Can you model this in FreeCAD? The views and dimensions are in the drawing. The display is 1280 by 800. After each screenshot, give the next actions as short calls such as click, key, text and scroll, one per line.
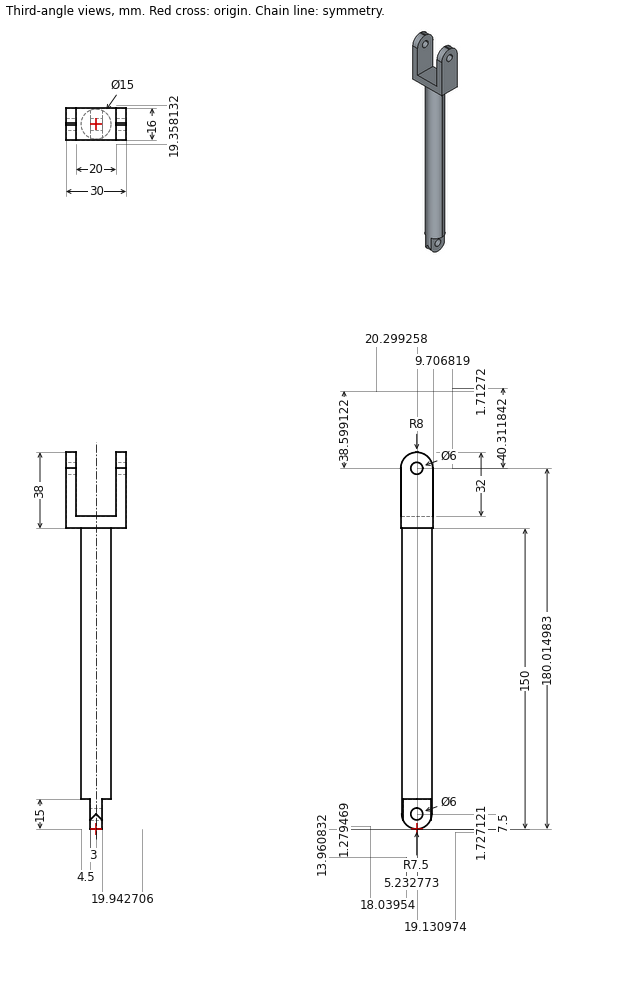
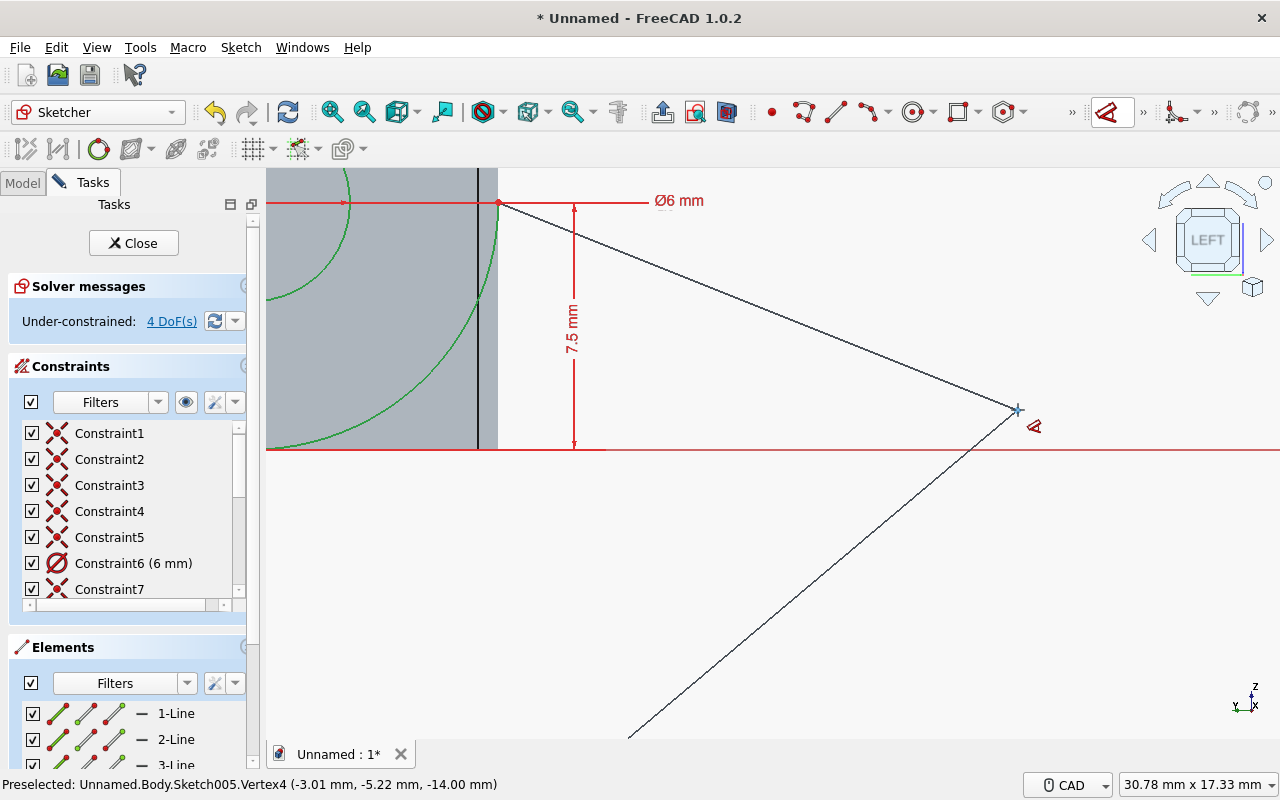
click(1017, 410)
click(1051, 430)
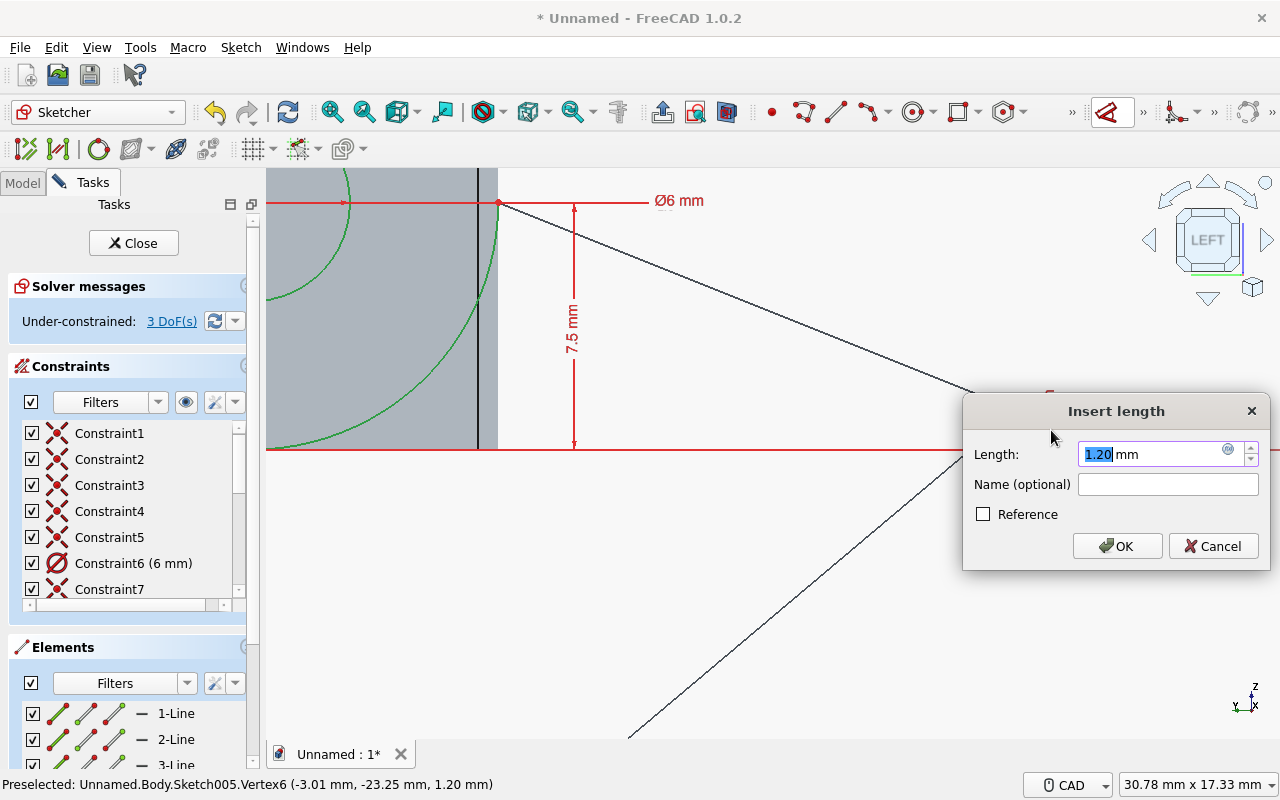
text(1.279469)
key(Return)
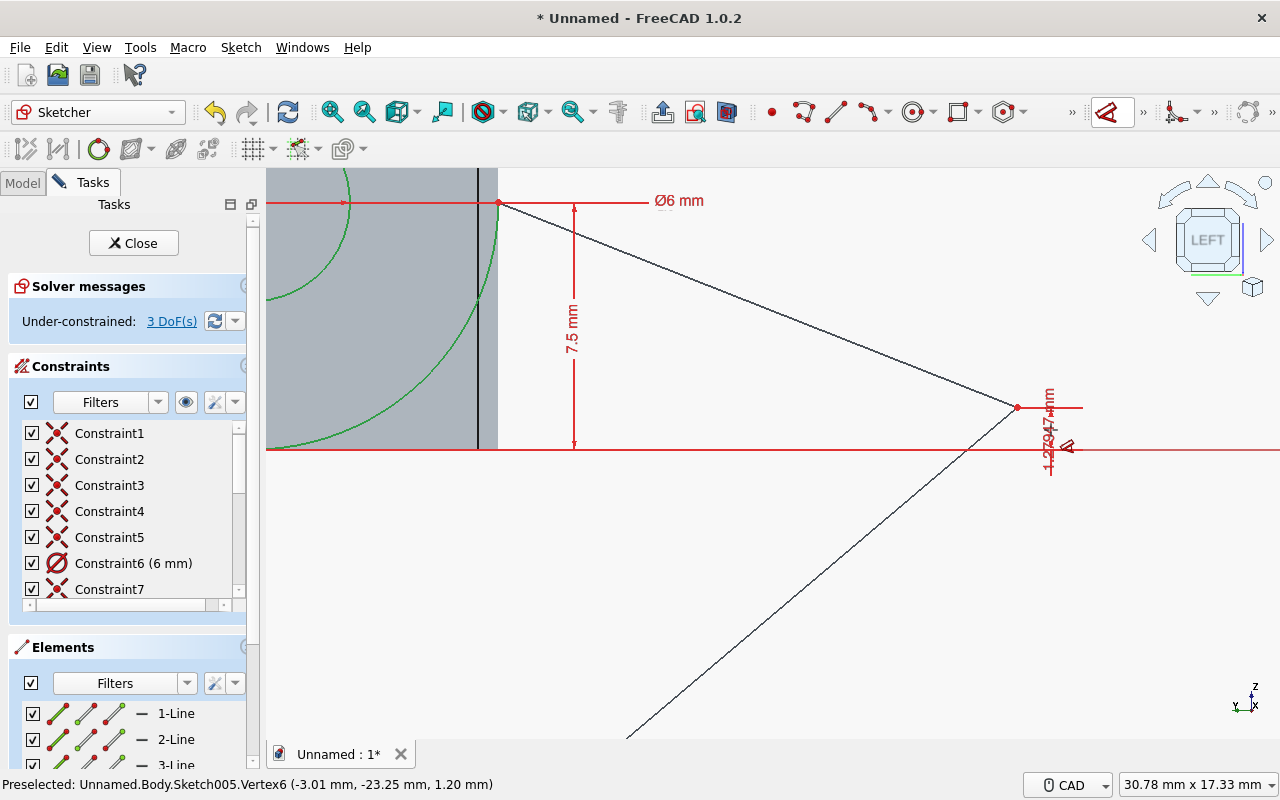
click(839, 559)
click(720, 374)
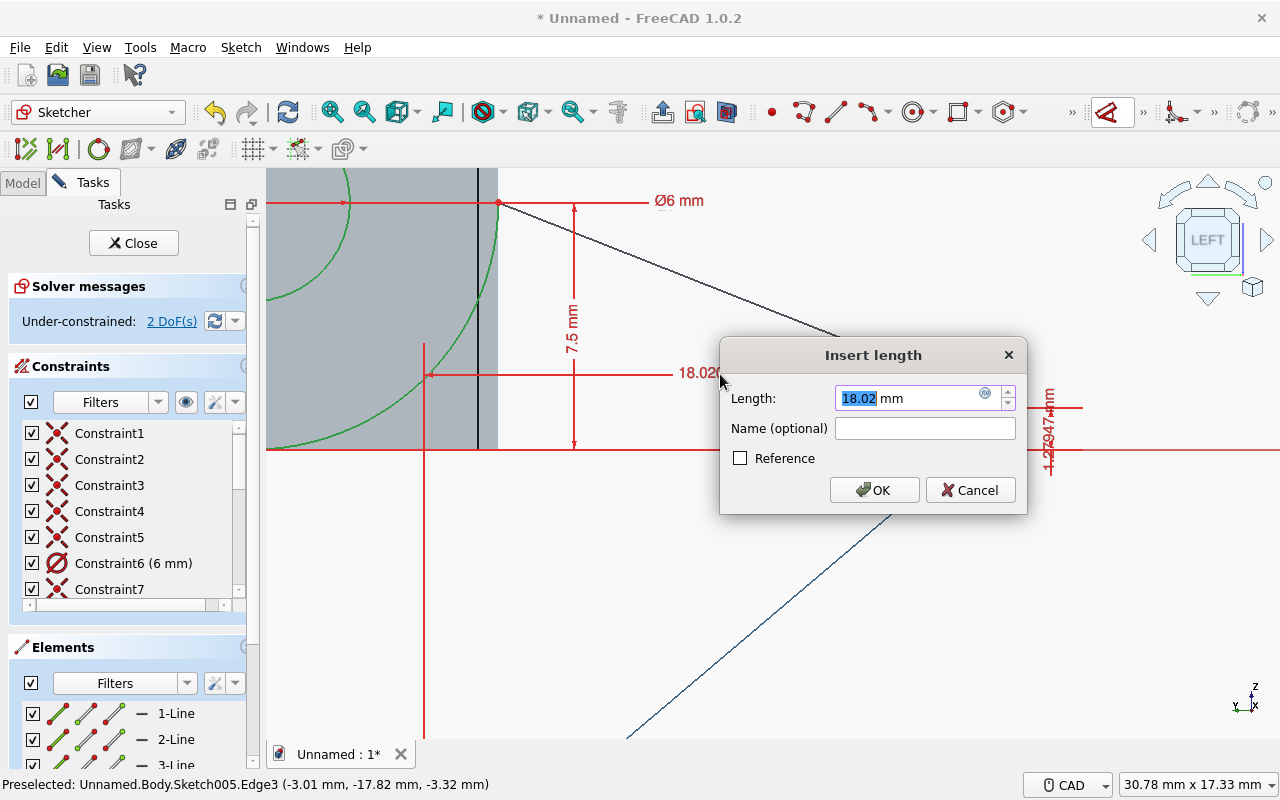
text(18.03954)
key(Return)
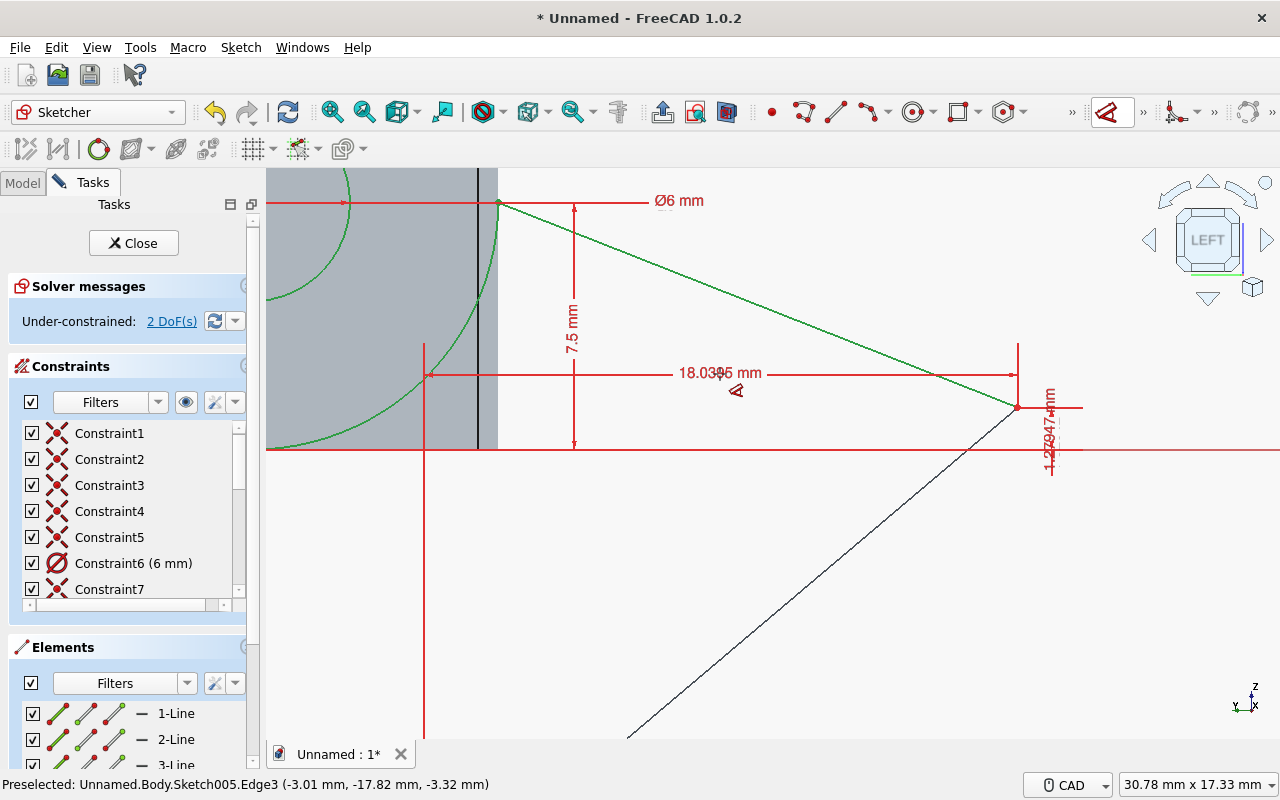
scroll(1019, 410, down, 4)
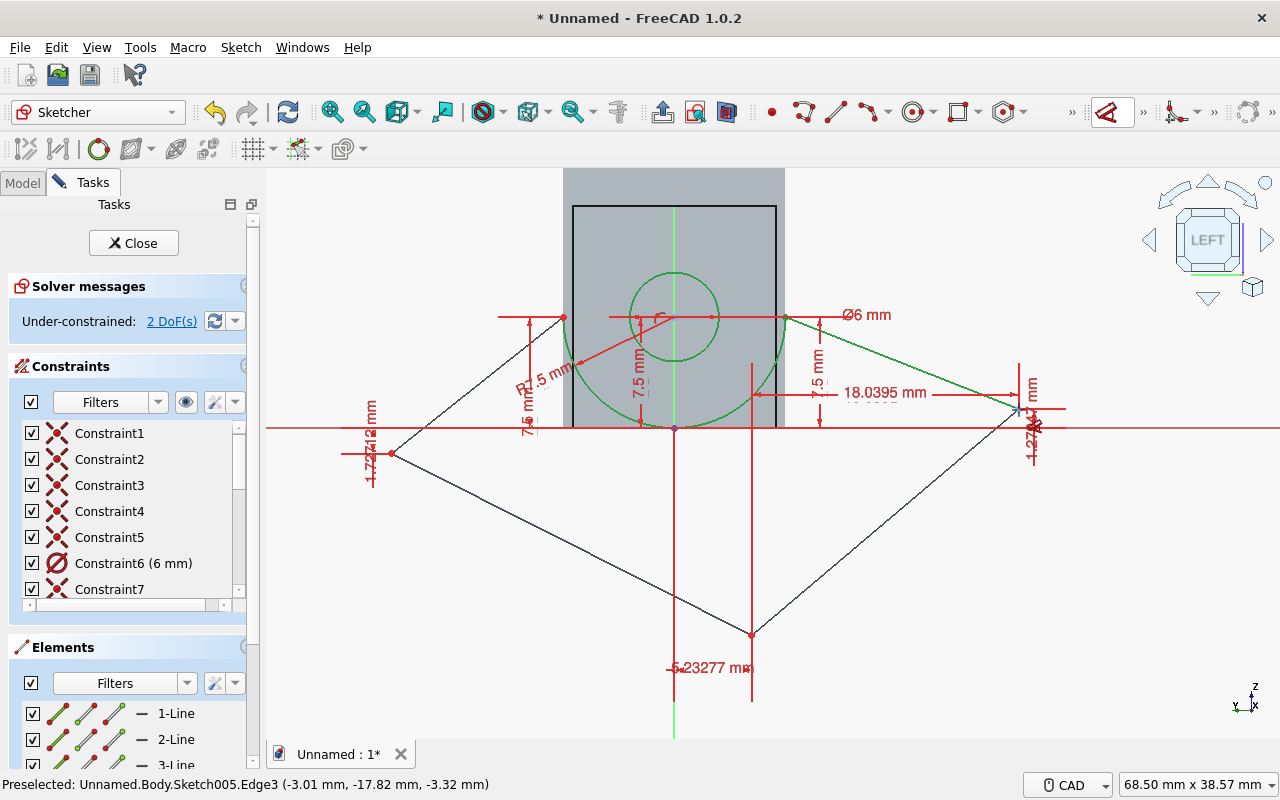
click(392, 454)
click(434, 394)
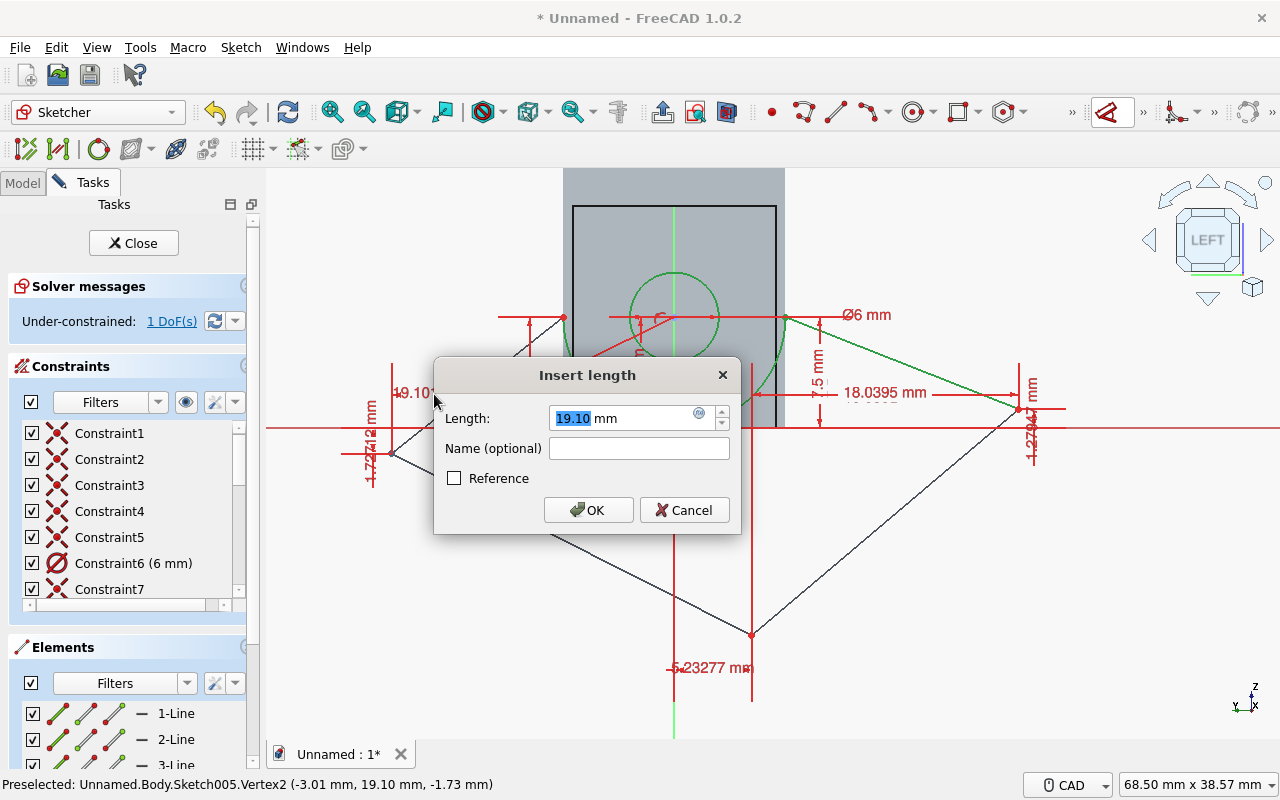
text(19.130974)
key(Return)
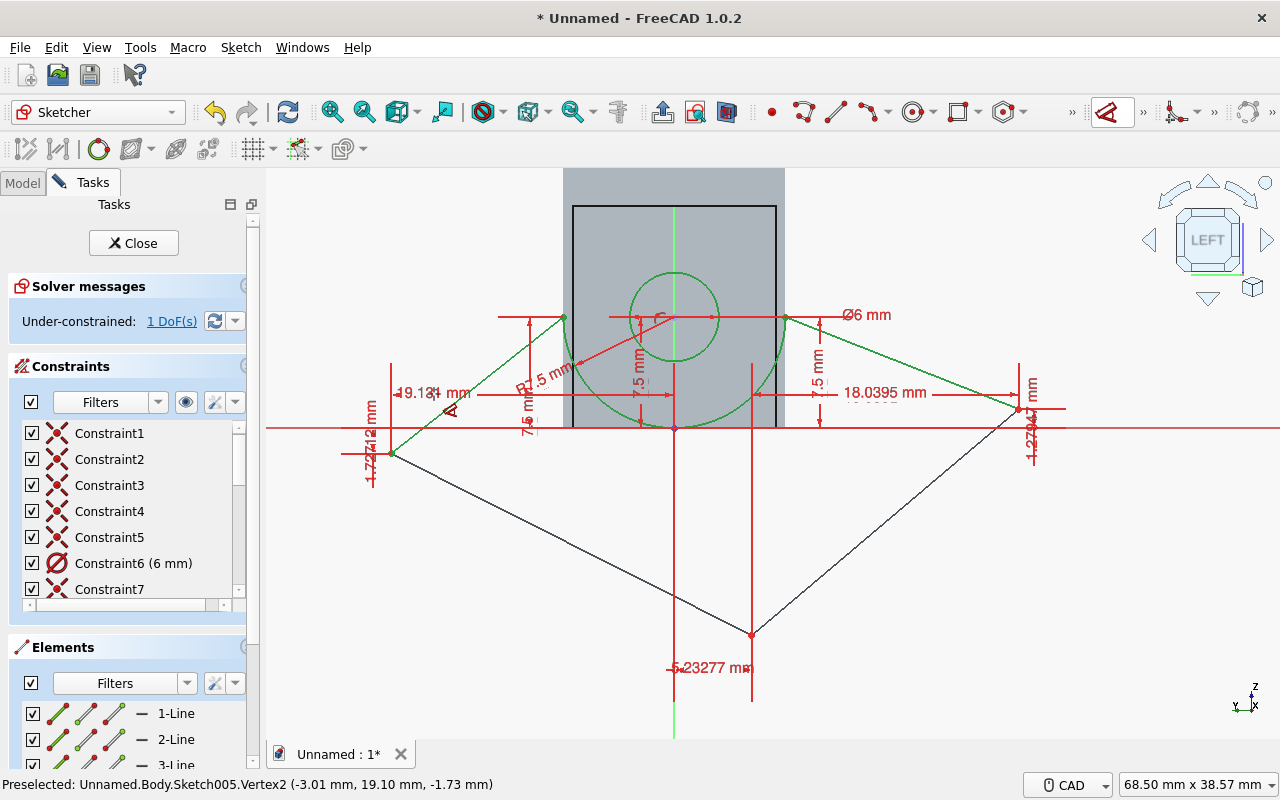
click(752, 635)
click(786, 532)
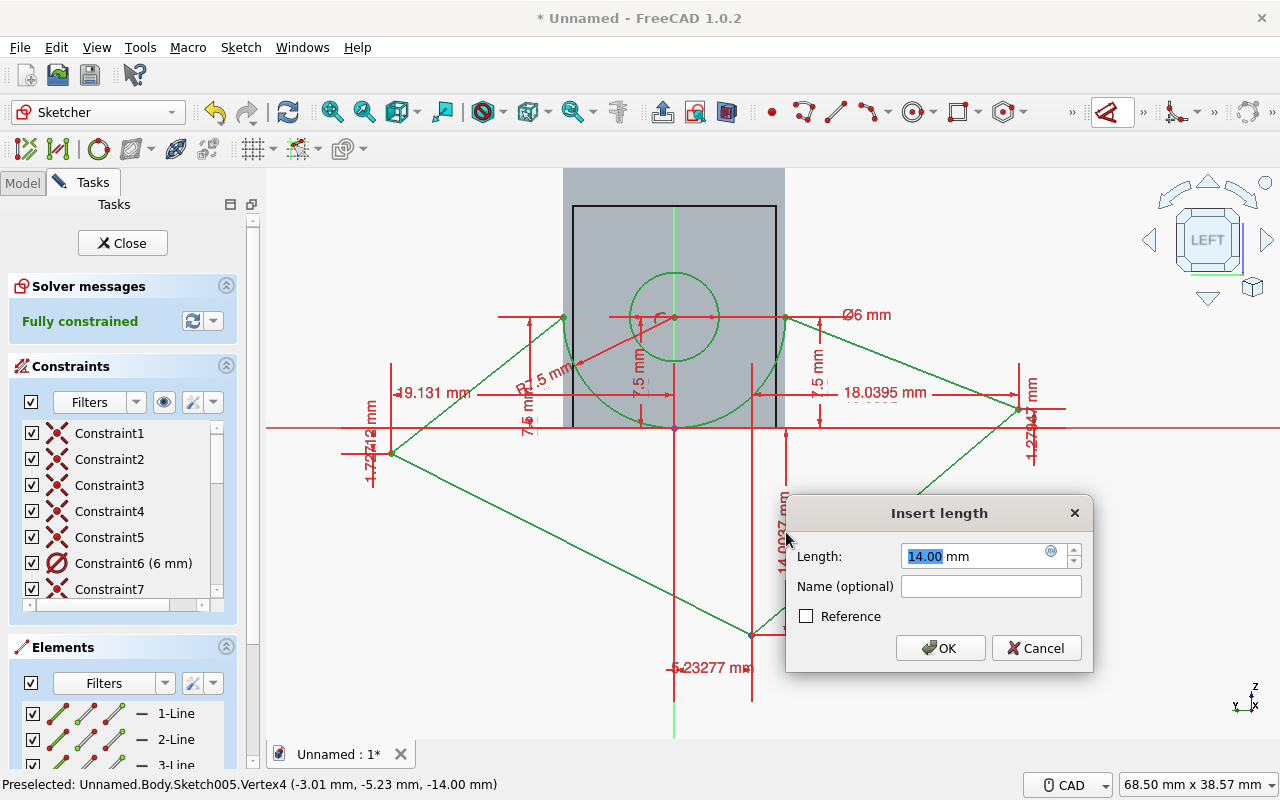
text(13.960832)
key(Return)
key(Escape)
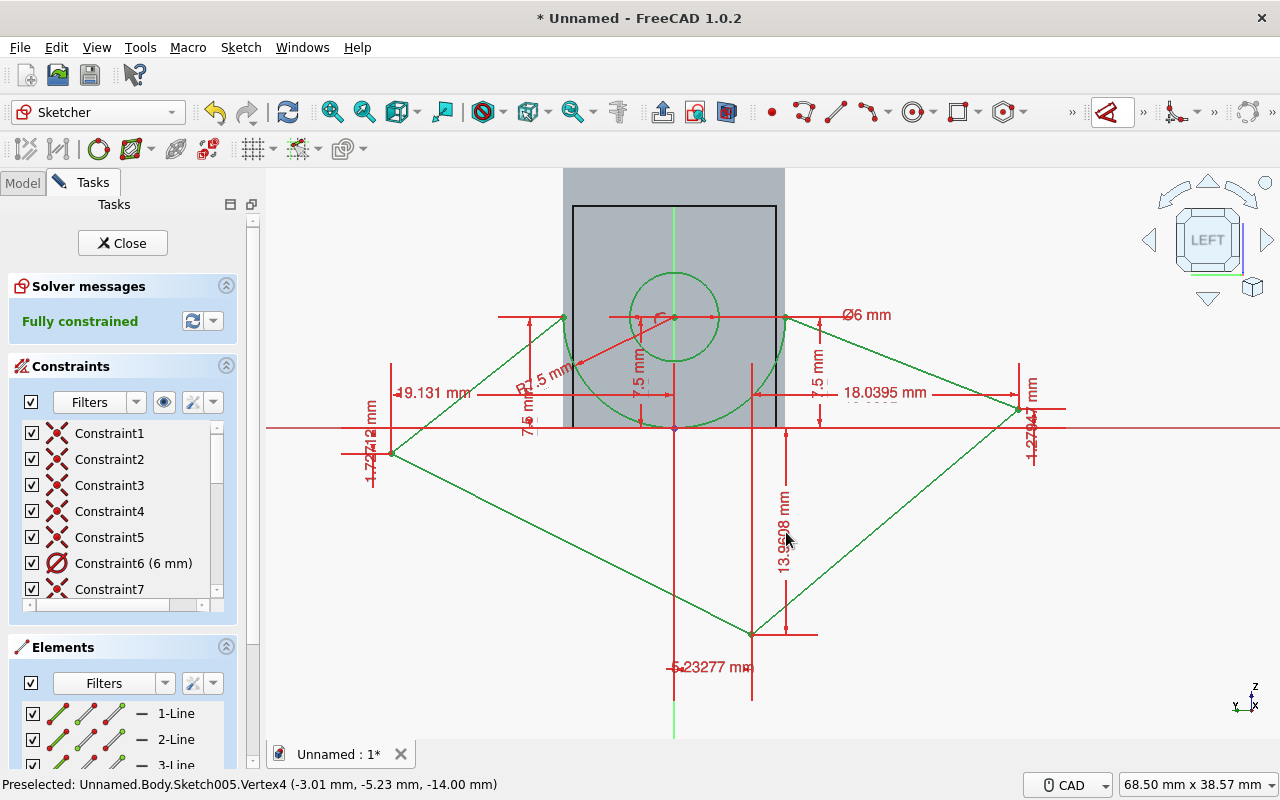
click(123, 243)